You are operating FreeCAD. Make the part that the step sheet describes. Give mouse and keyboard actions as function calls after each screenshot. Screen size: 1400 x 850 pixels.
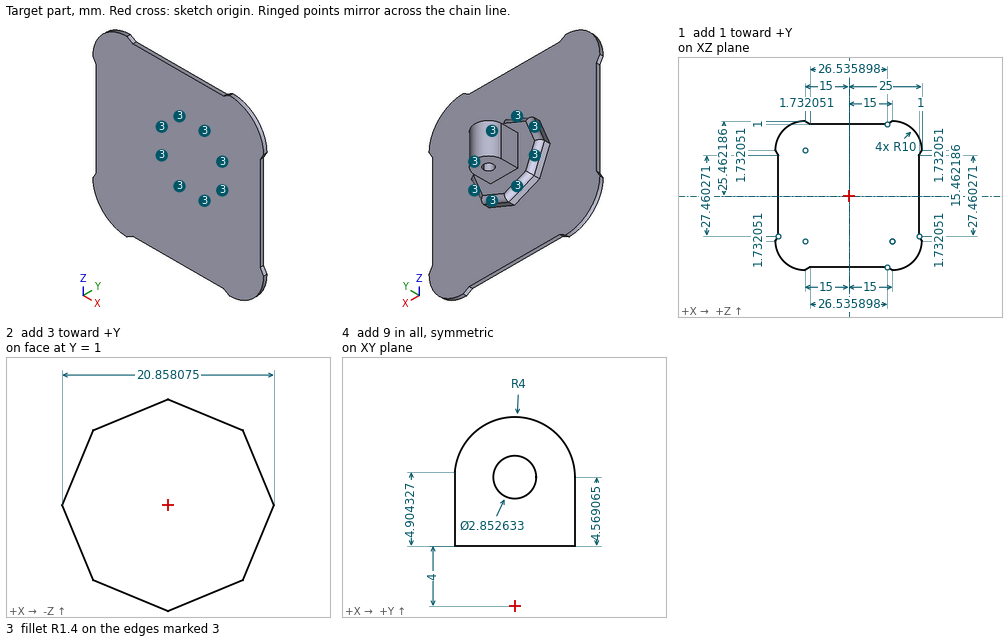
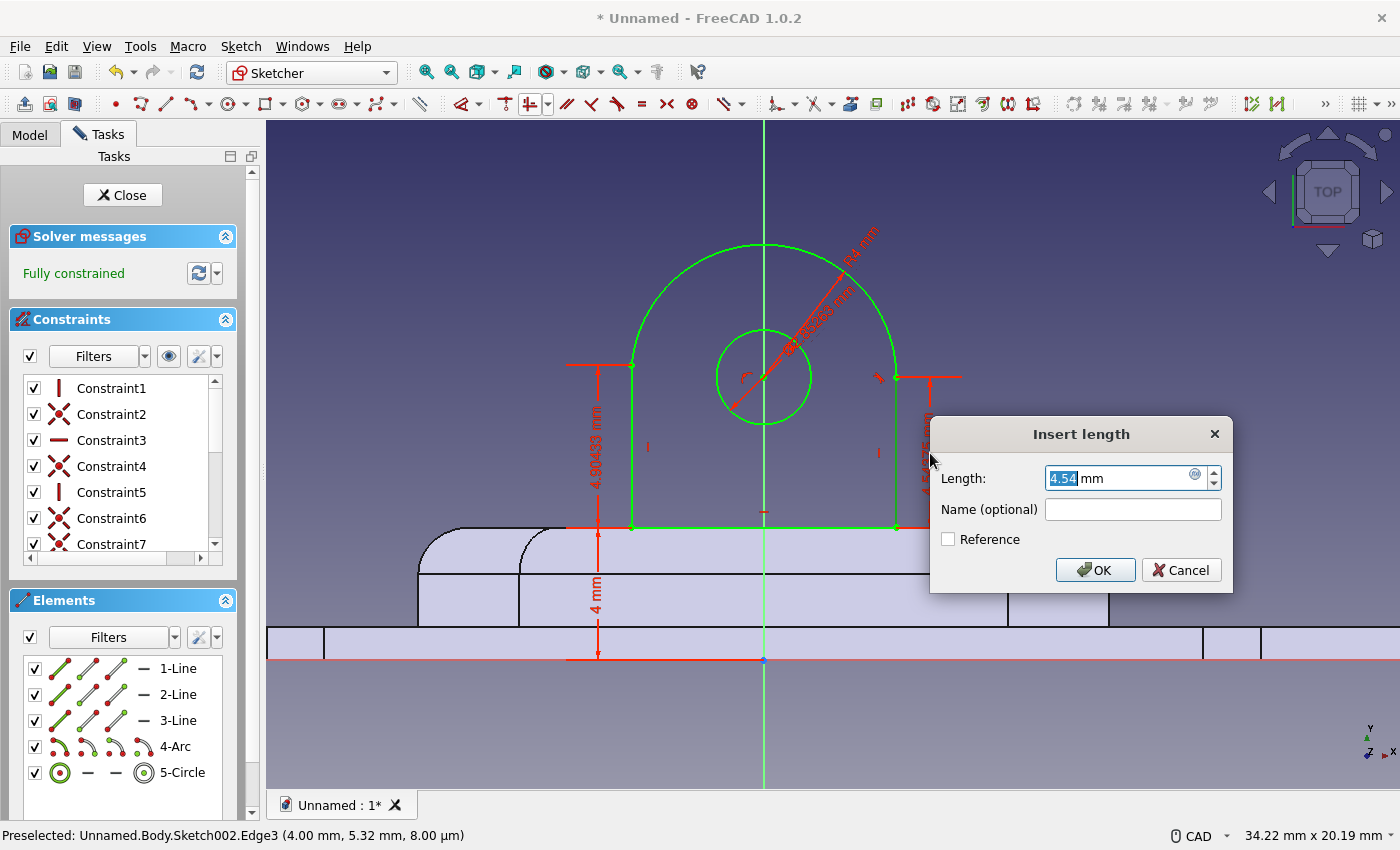
text(4.569065)
key(Return)
key(Escape)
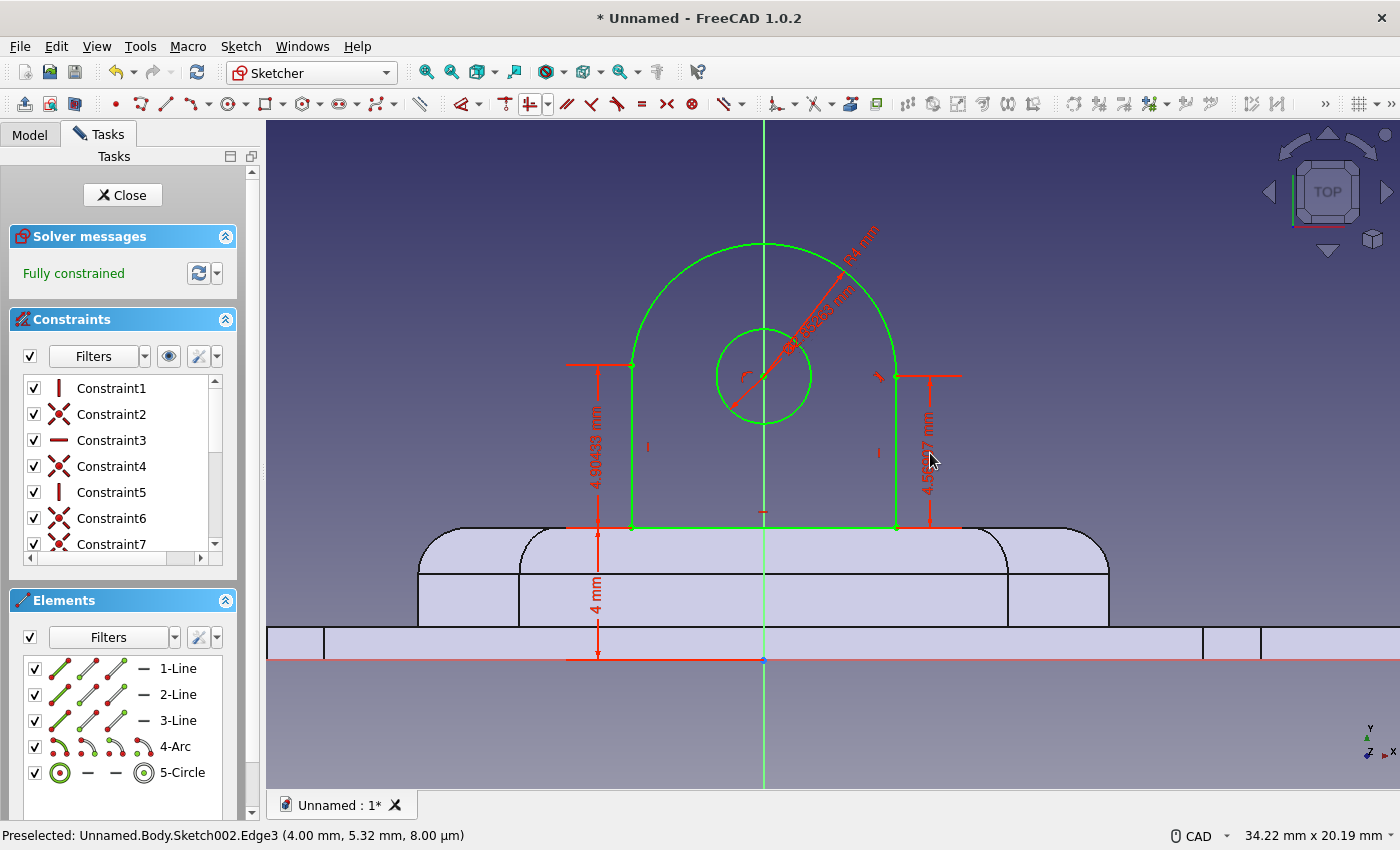
click(123, 195)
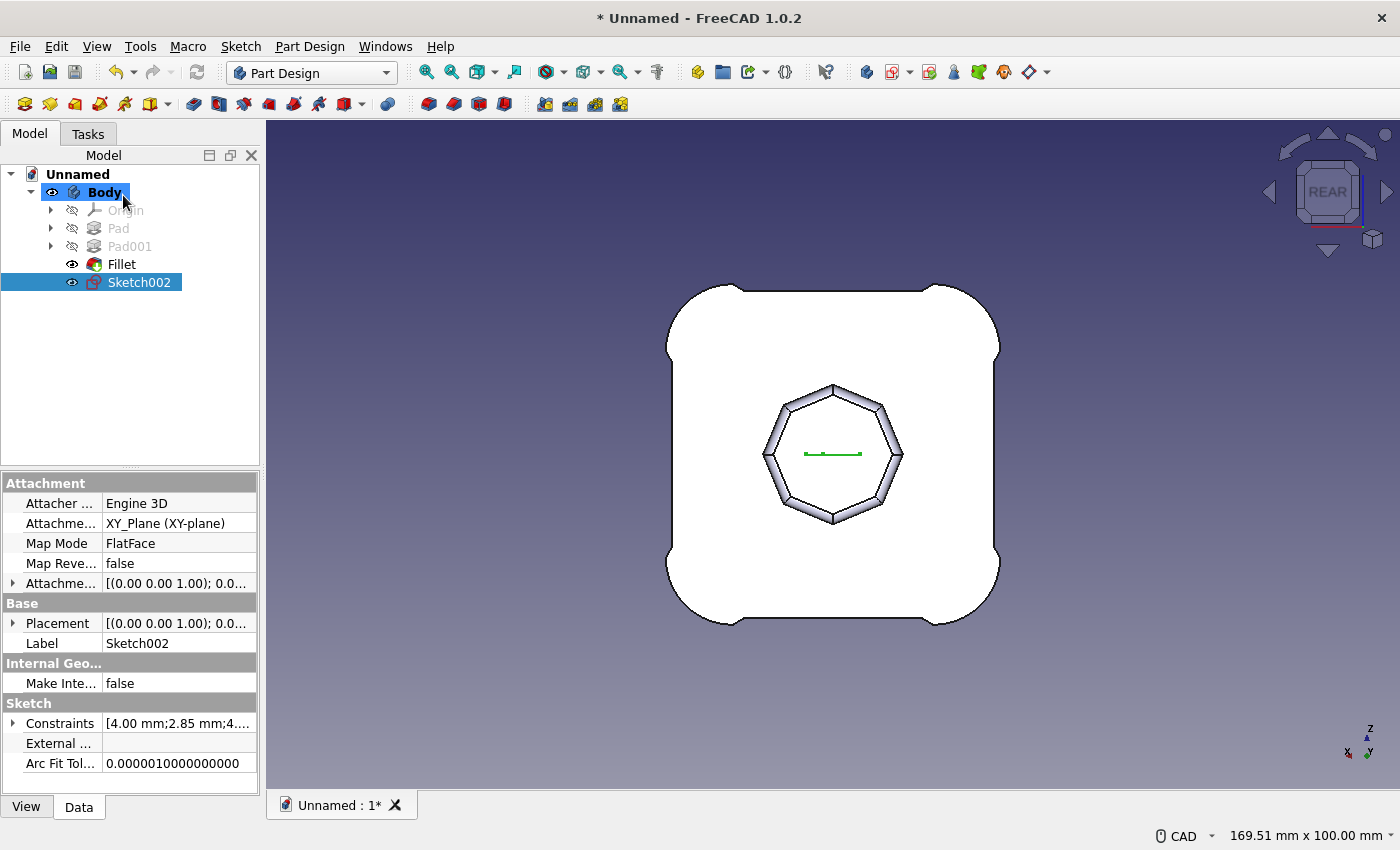
click(25, 104)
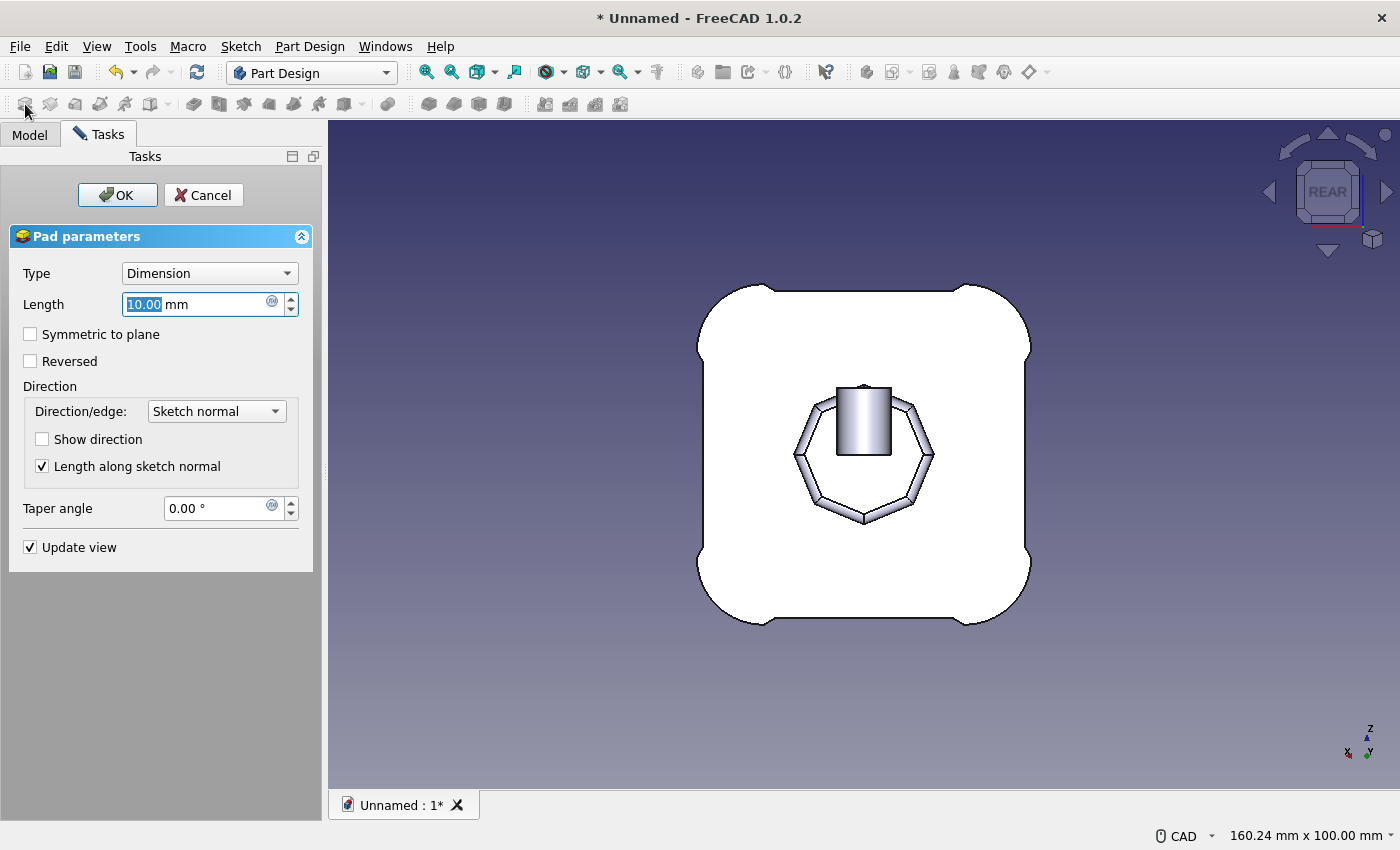
text(9)
key(Tab)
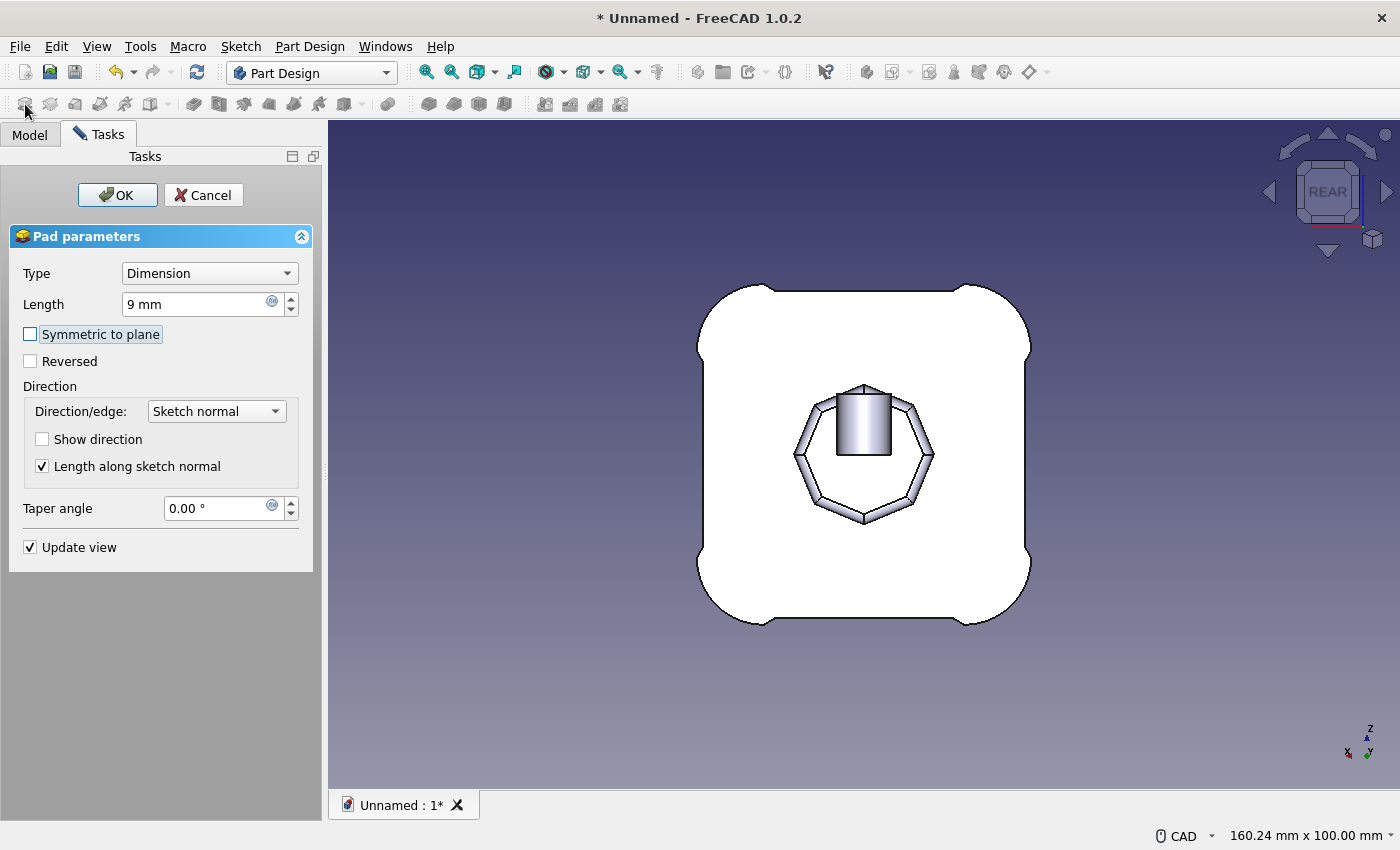
click(31, 334)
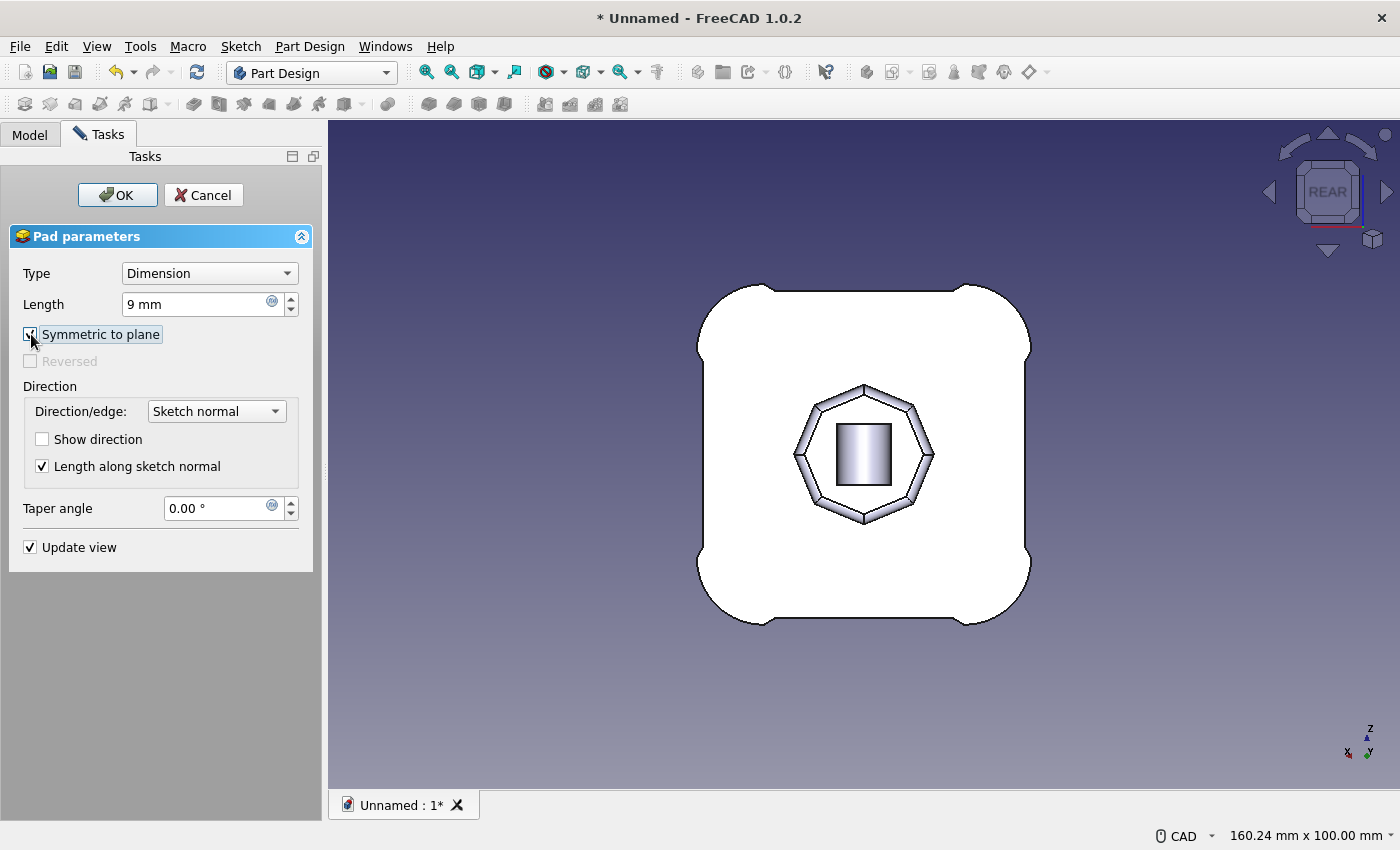
click(118, 195)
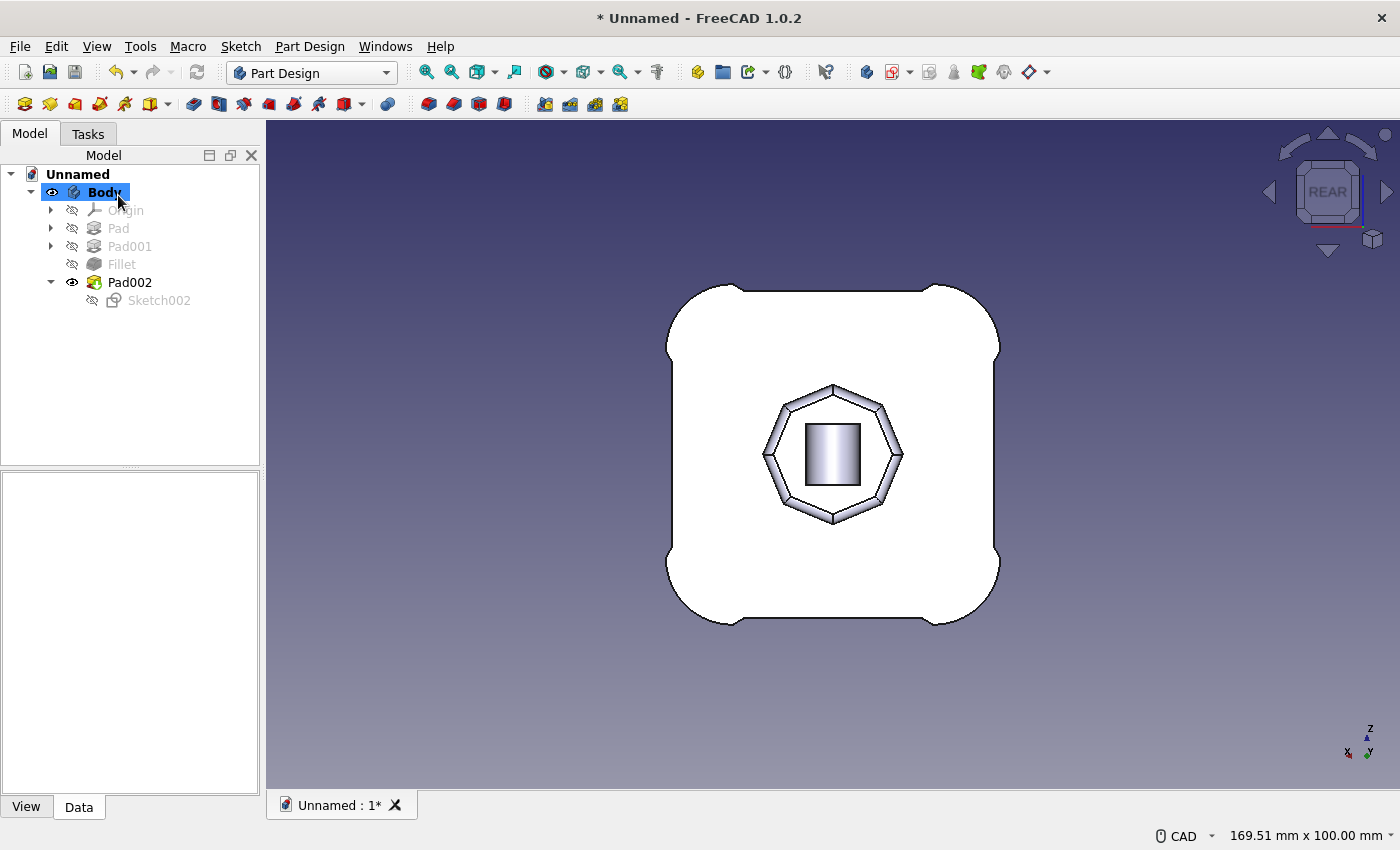
key(0)